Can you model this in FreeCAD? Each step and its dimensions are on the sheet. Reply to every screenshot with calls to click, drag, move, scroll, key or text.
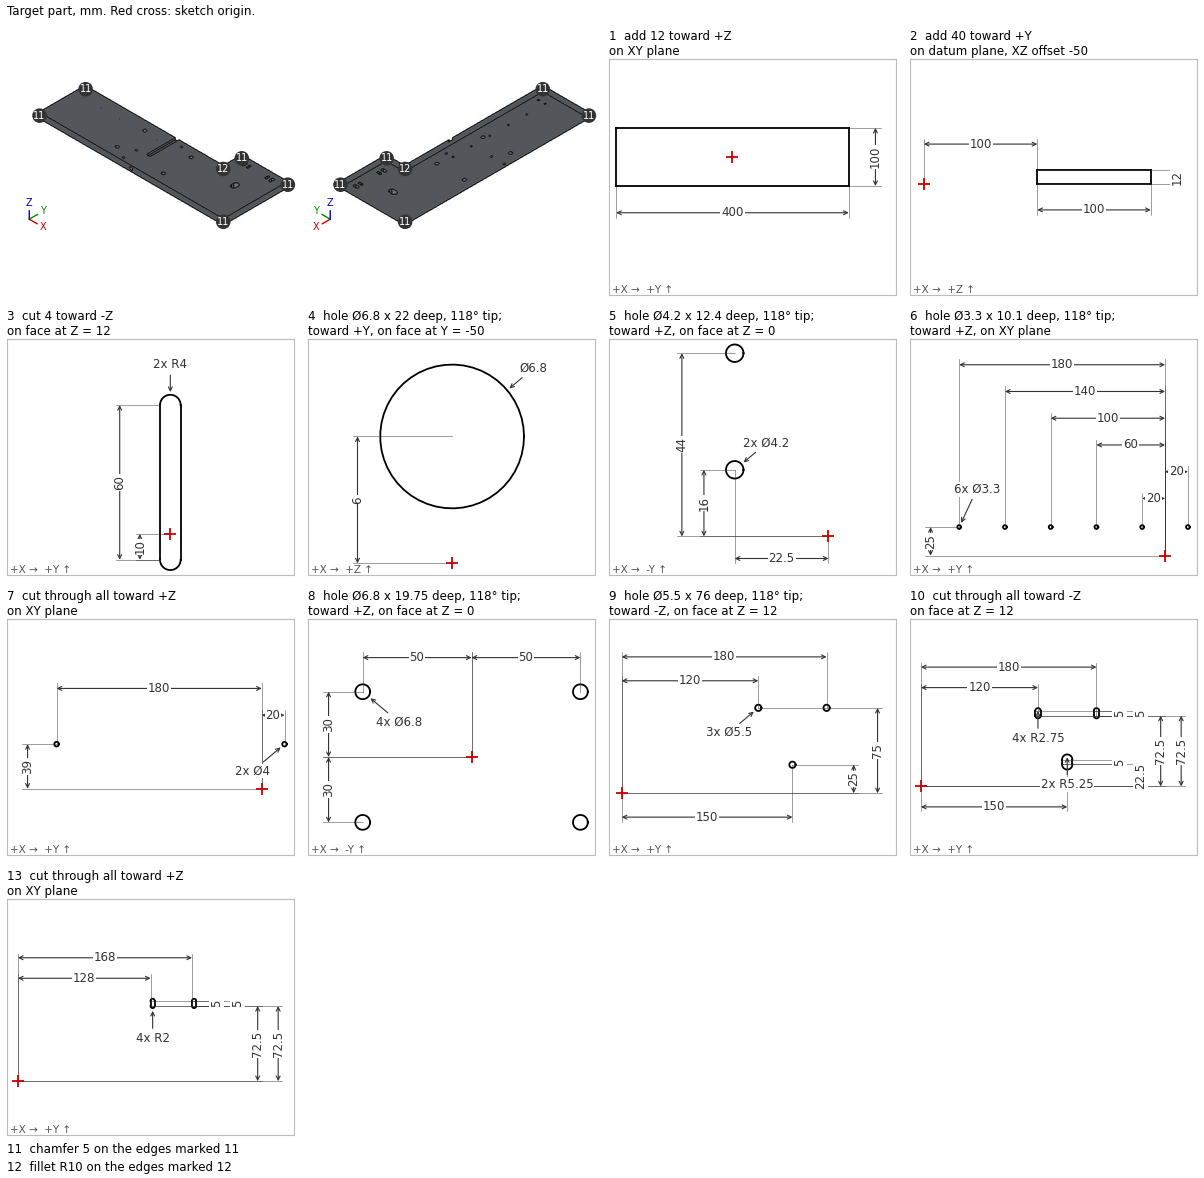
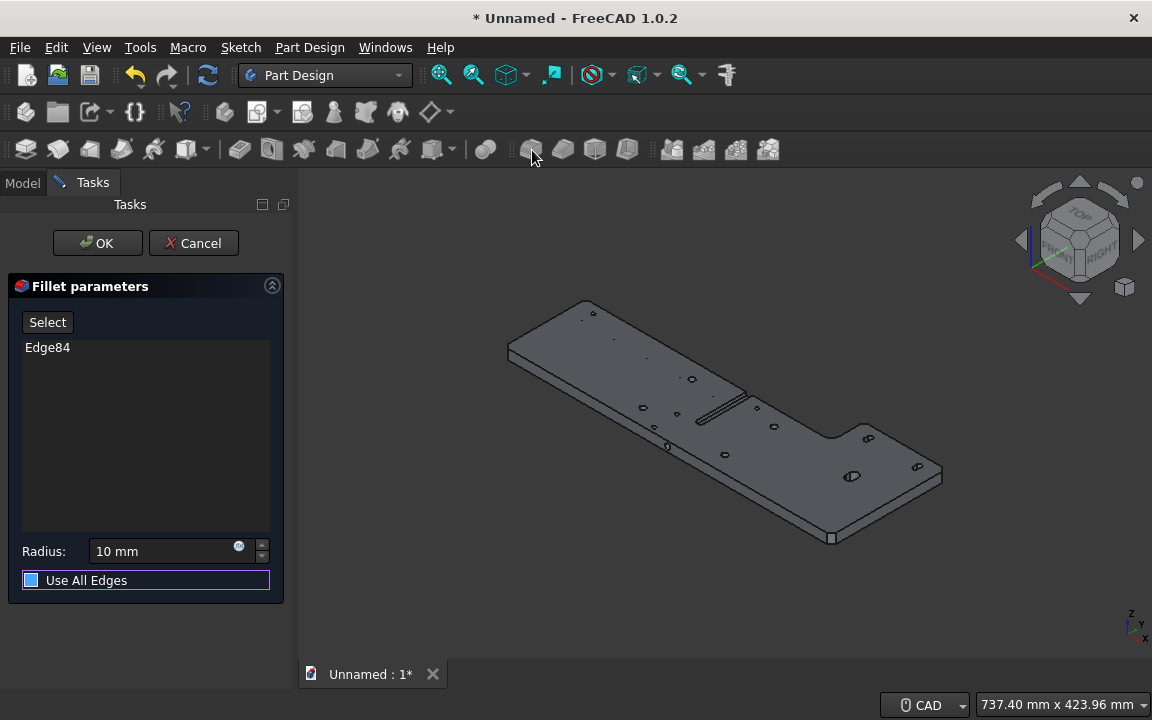
click(98, 243)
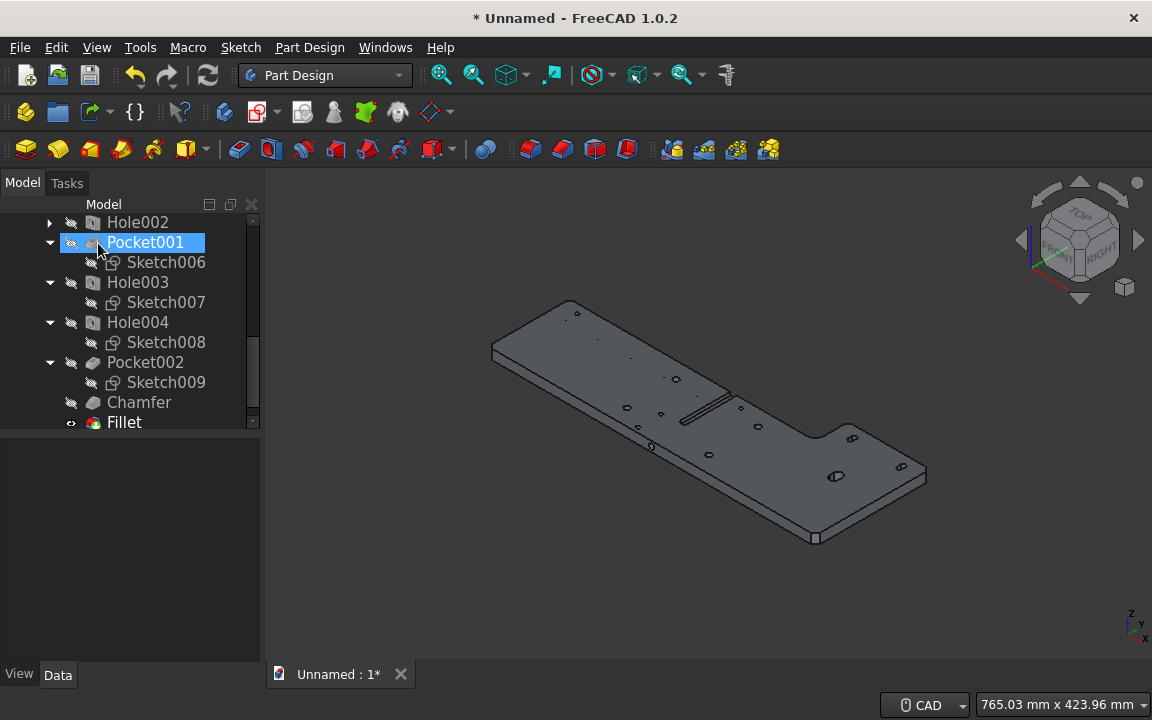
click(258, 112)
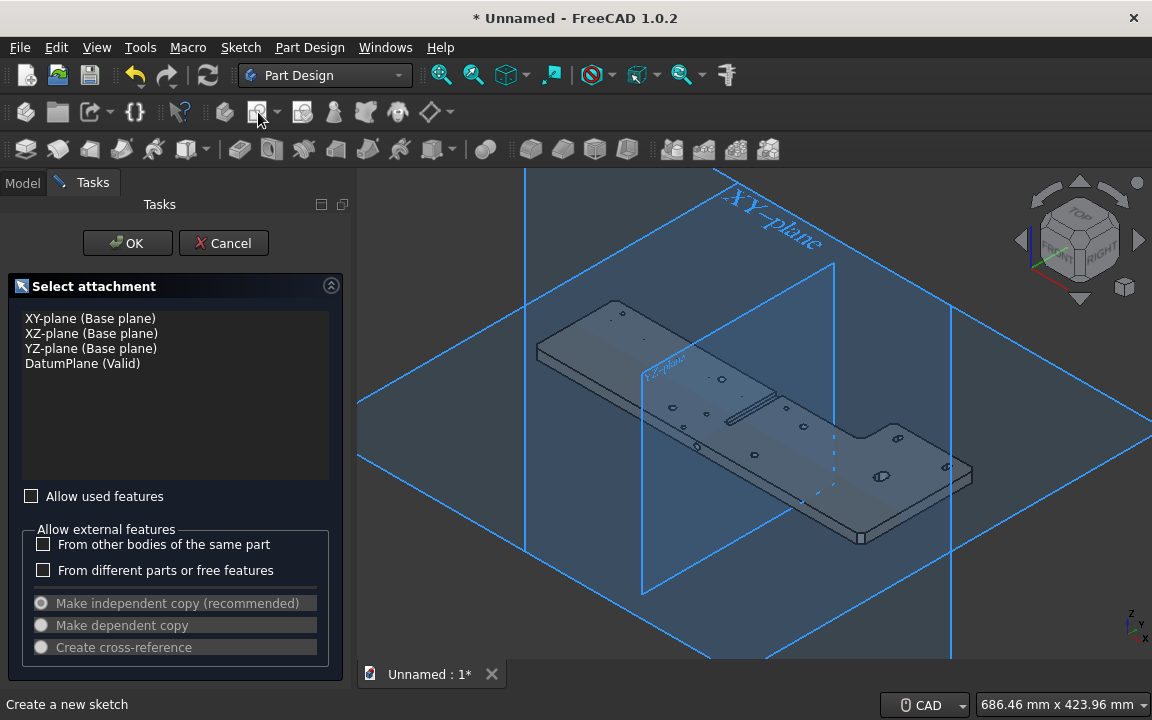
click(82, 318)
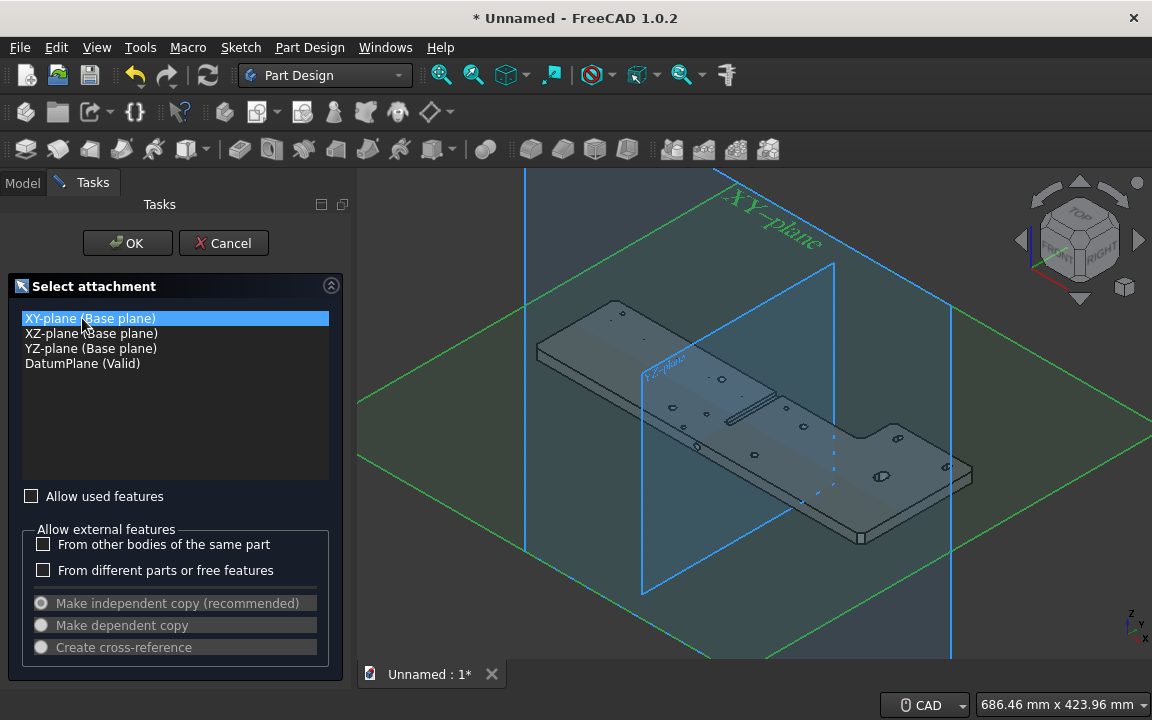
click(128, 243)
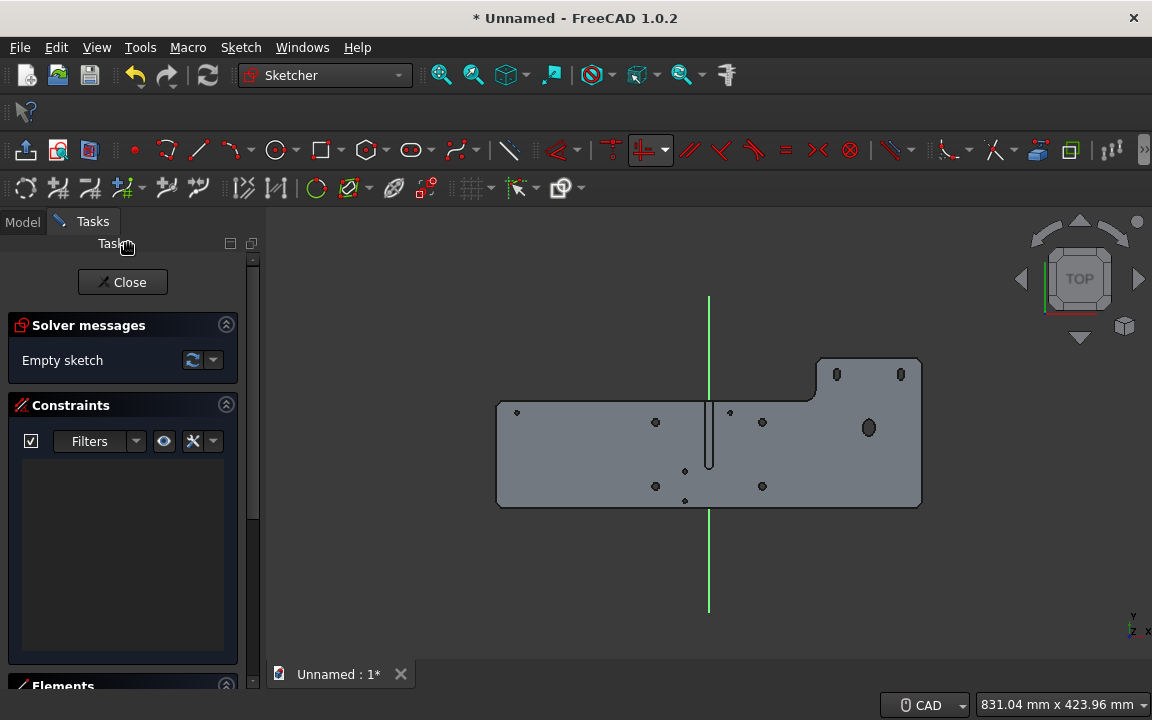
click(90, 150)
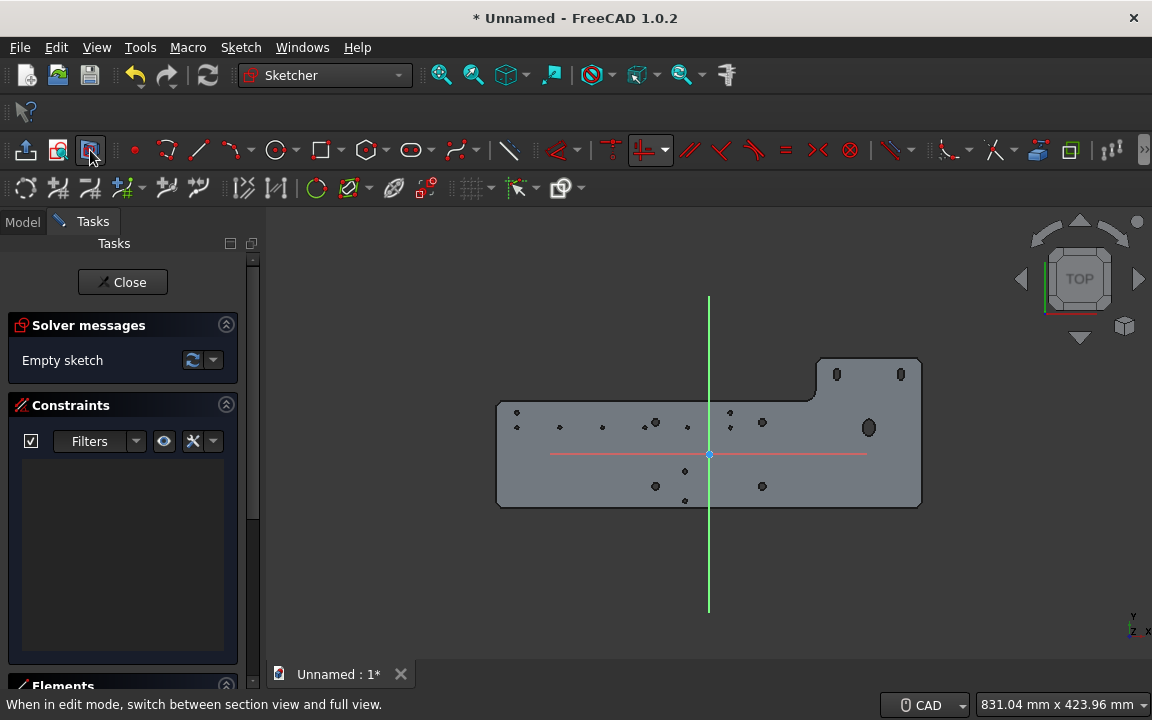
scroll(892, 369, up, 12)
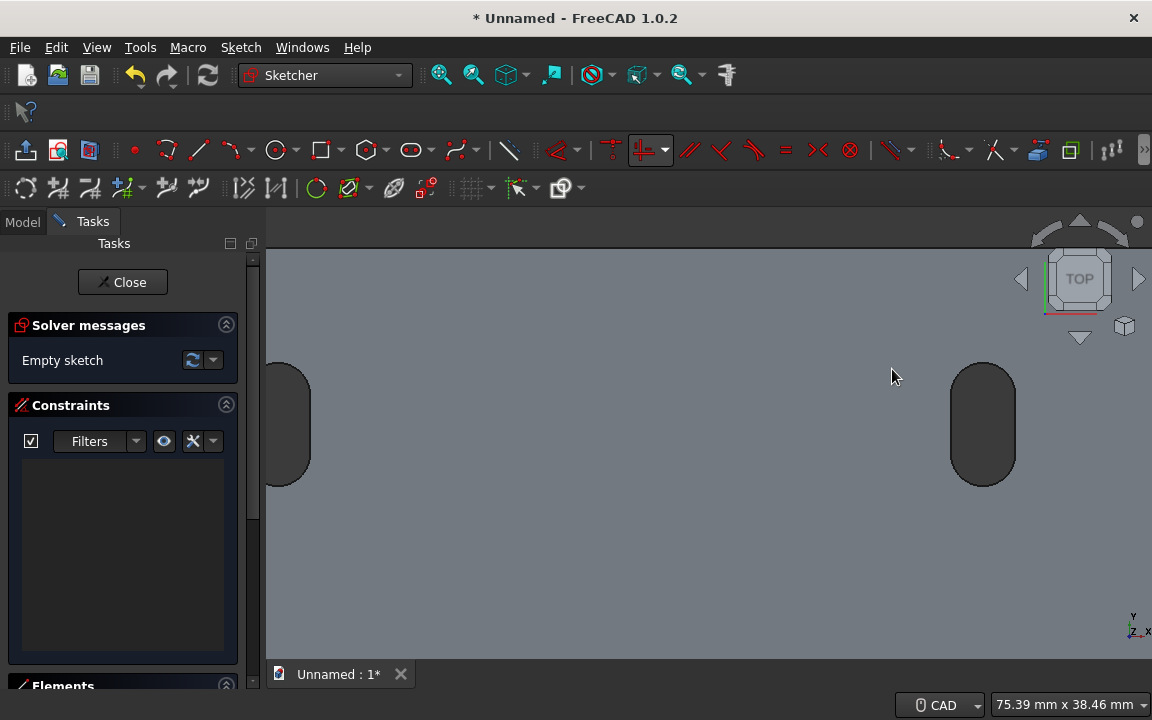
click(412, 150)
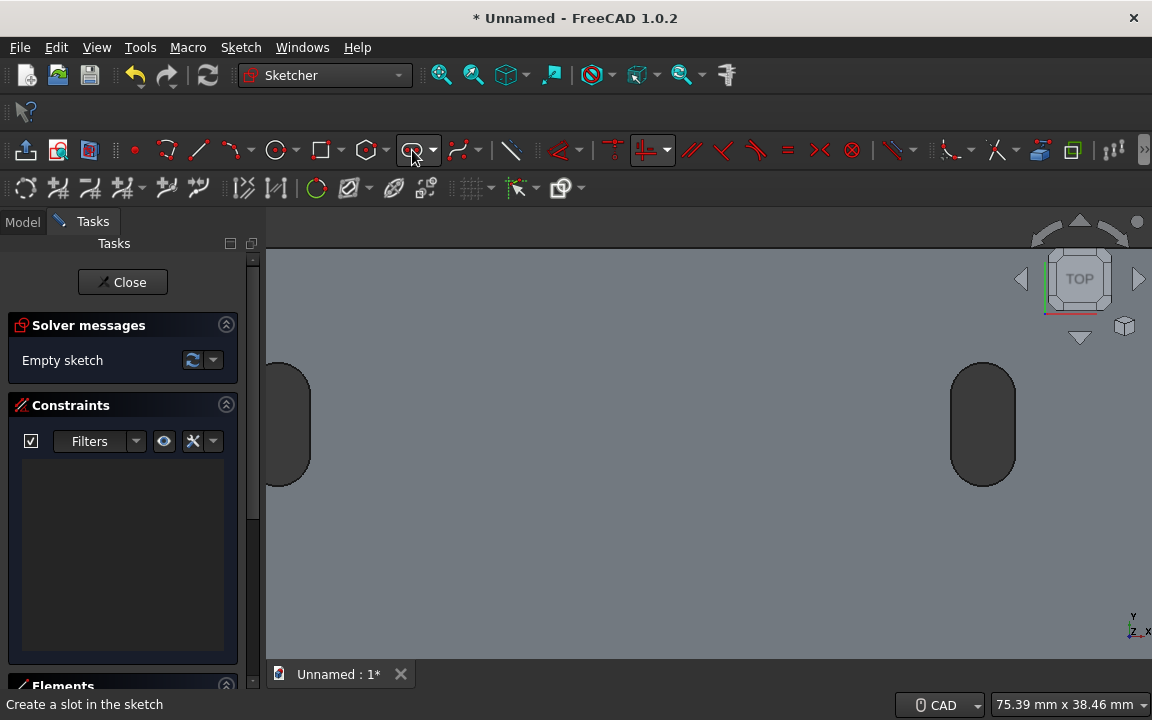
click(395, 454)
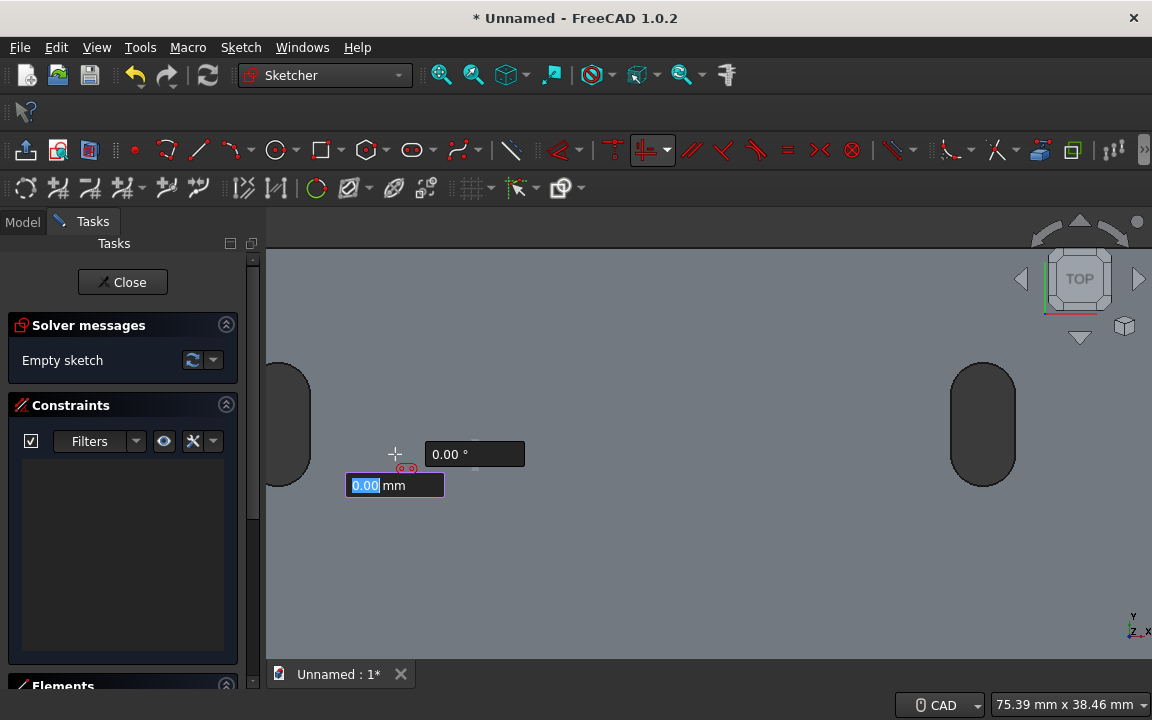
click(395, 395)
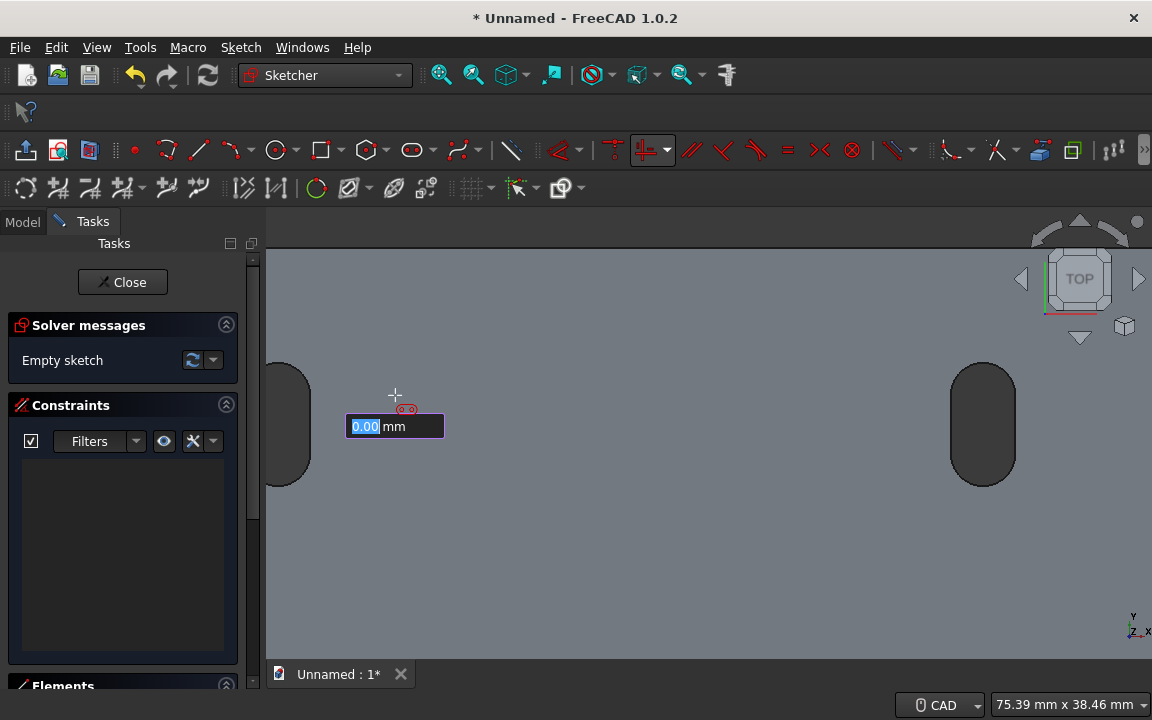
click(419, 425)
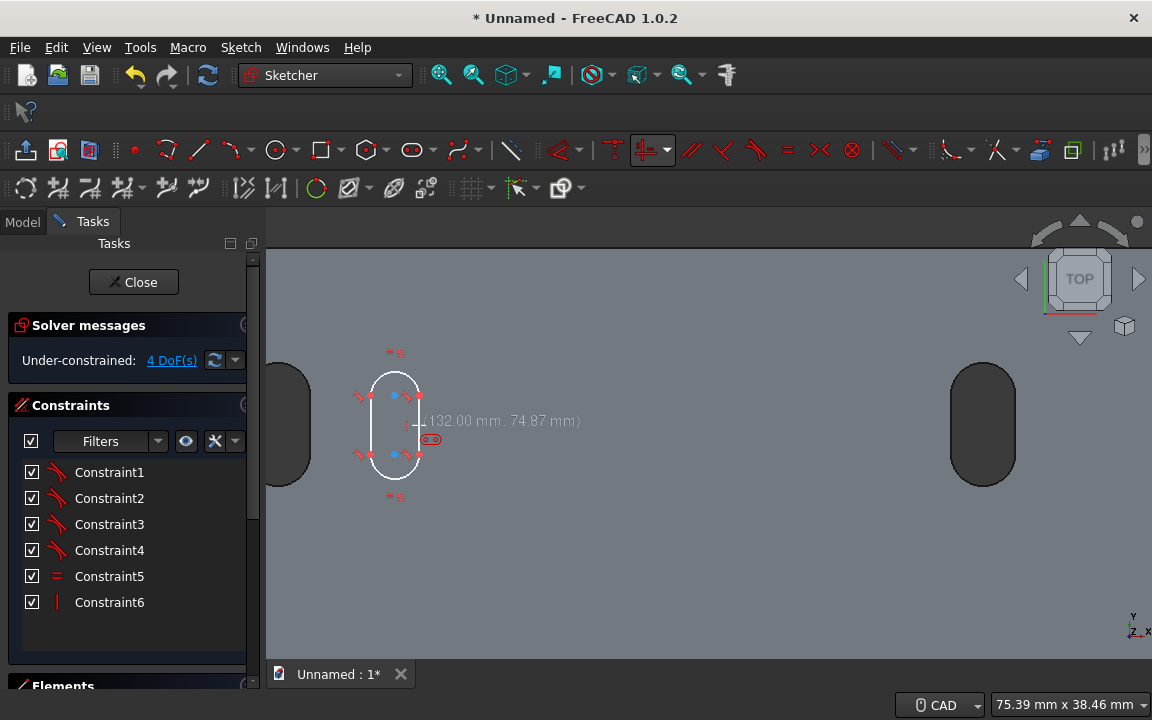
click(866, 454)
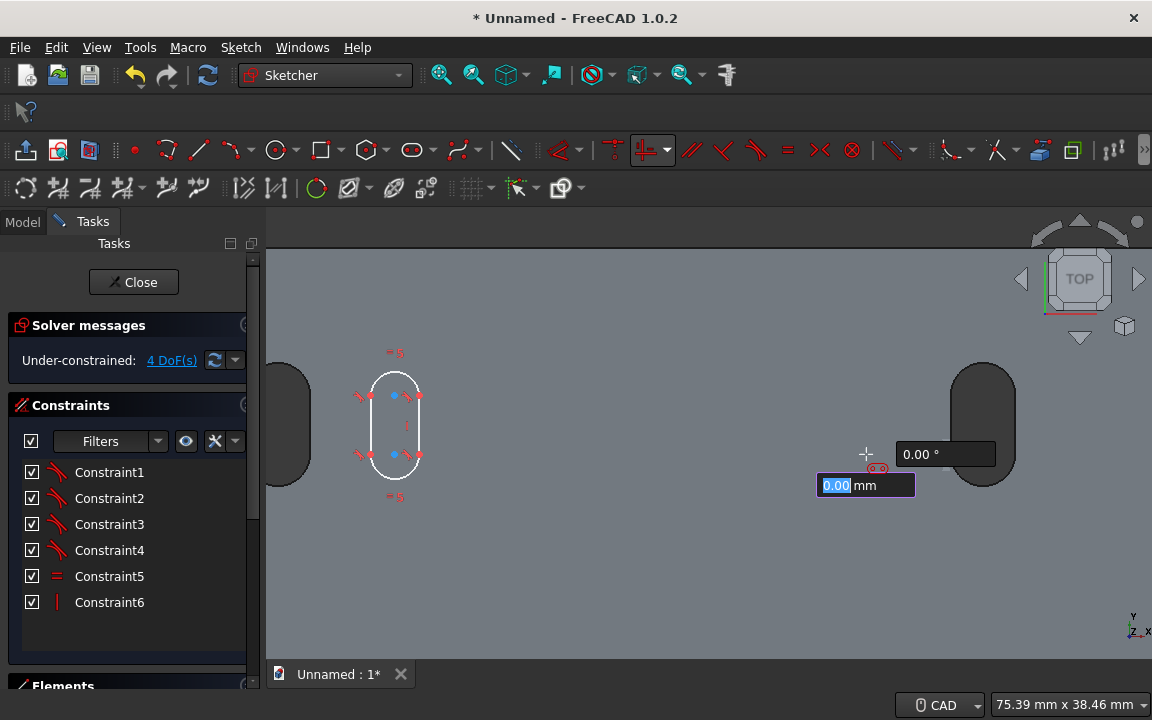
click(866, 395)